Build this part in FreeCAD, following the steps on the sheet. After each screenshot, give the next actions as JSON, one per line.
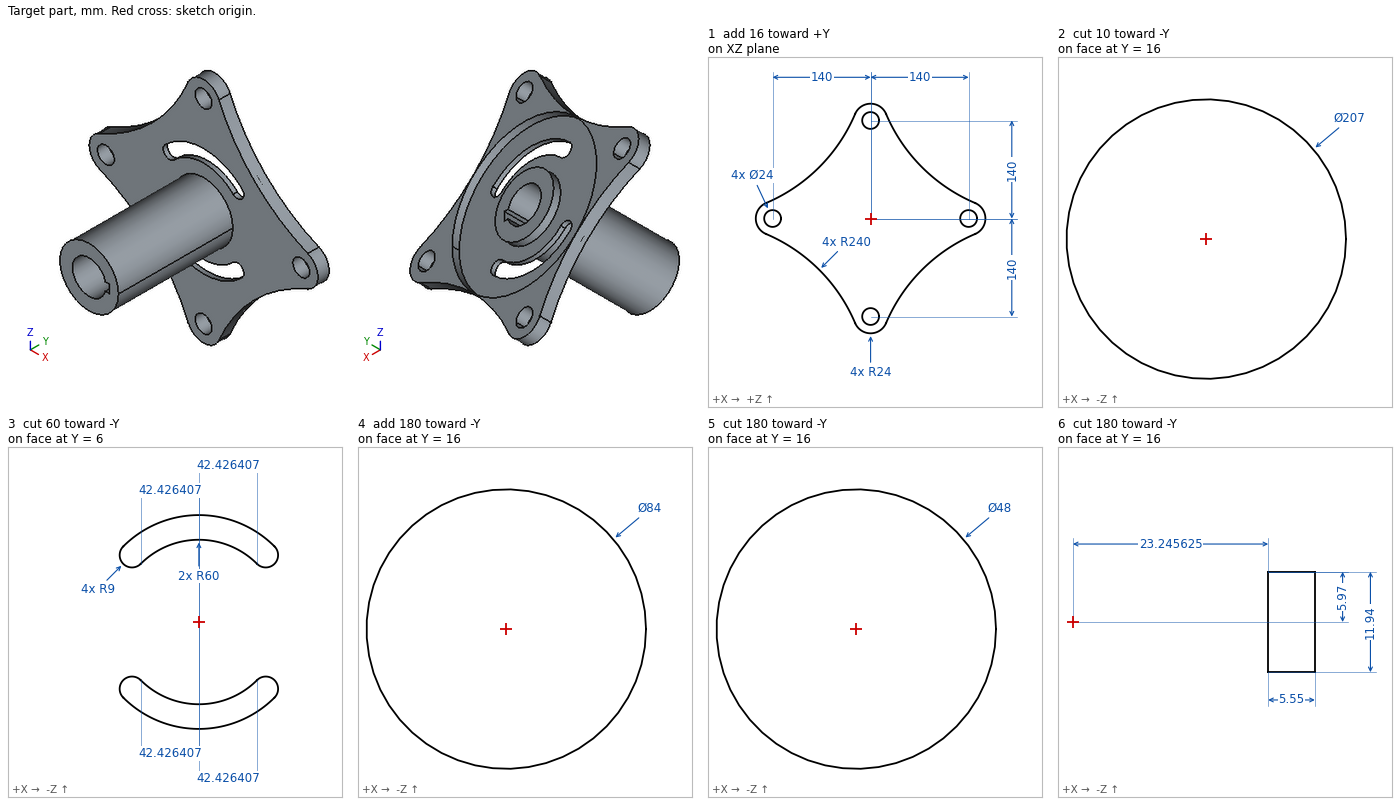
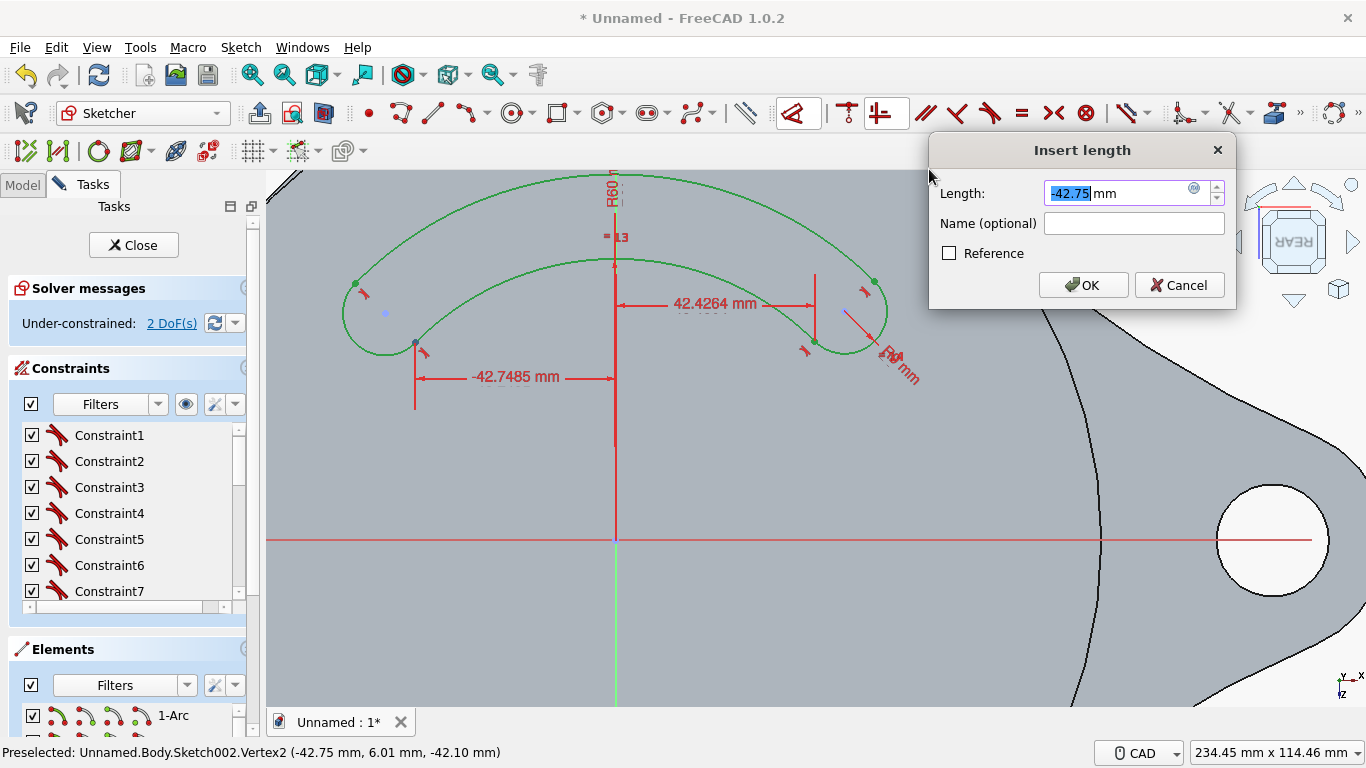
{"action": "type", "text": "-42.426407"}
{"action": "key", "text": "Return"}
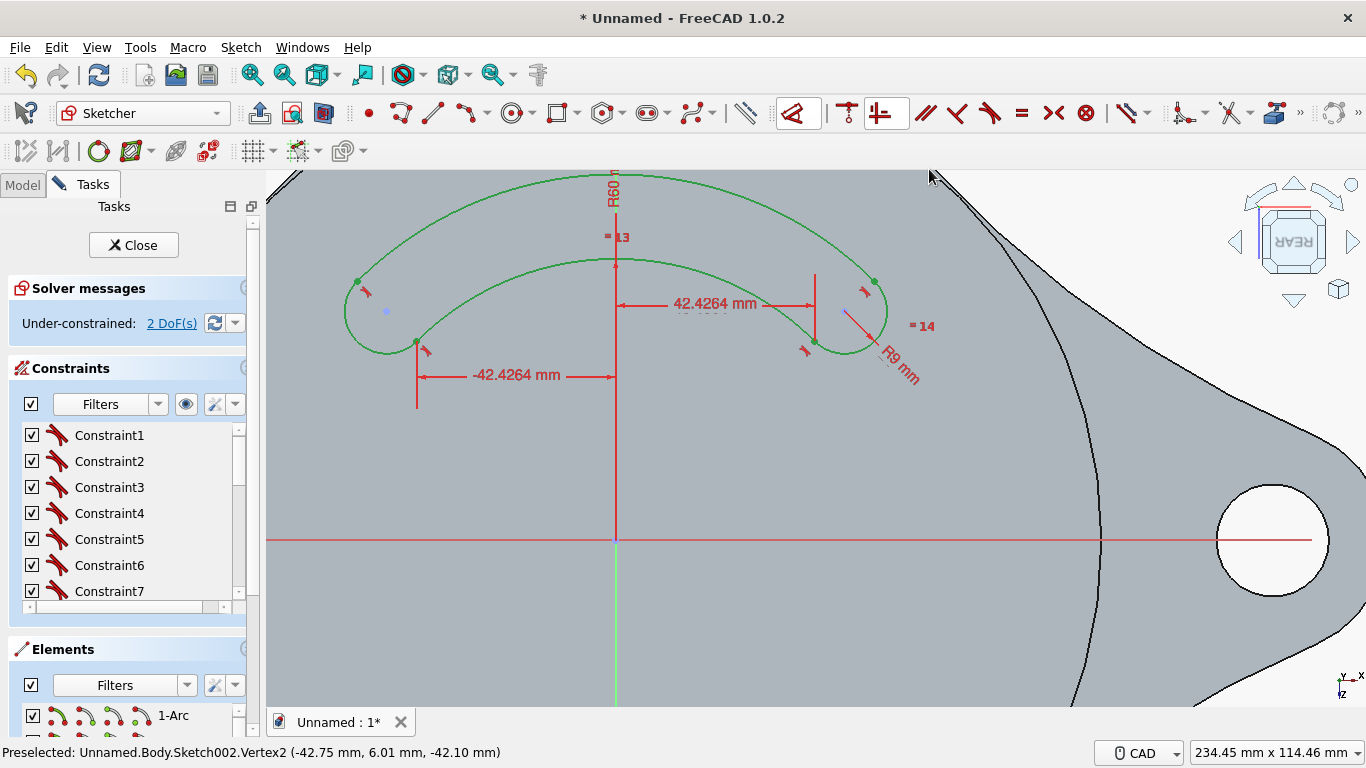
{"action": "scroll", "coordinate": [855, 355], "scroll_direction": "down", "scroll_amount": 4}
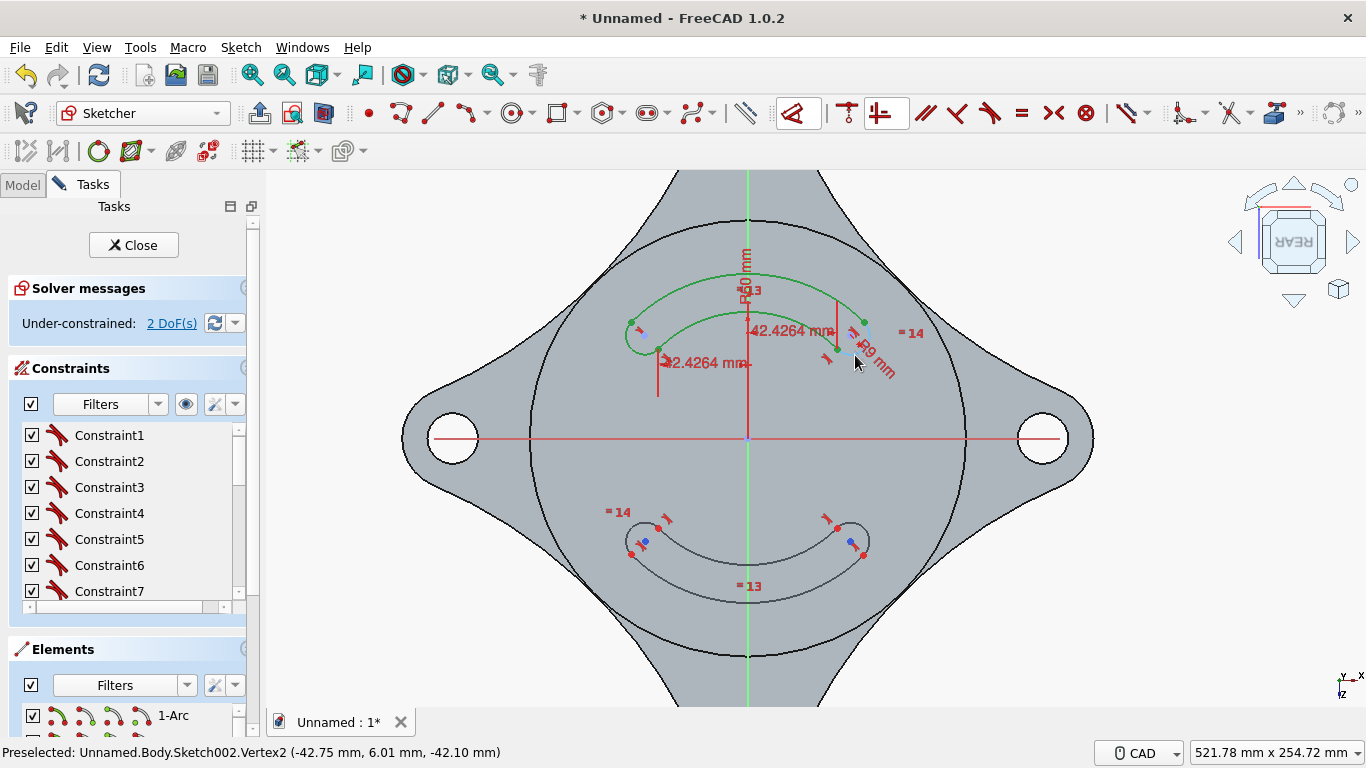
{"action": "left_click", "coordinate": [659, 528]}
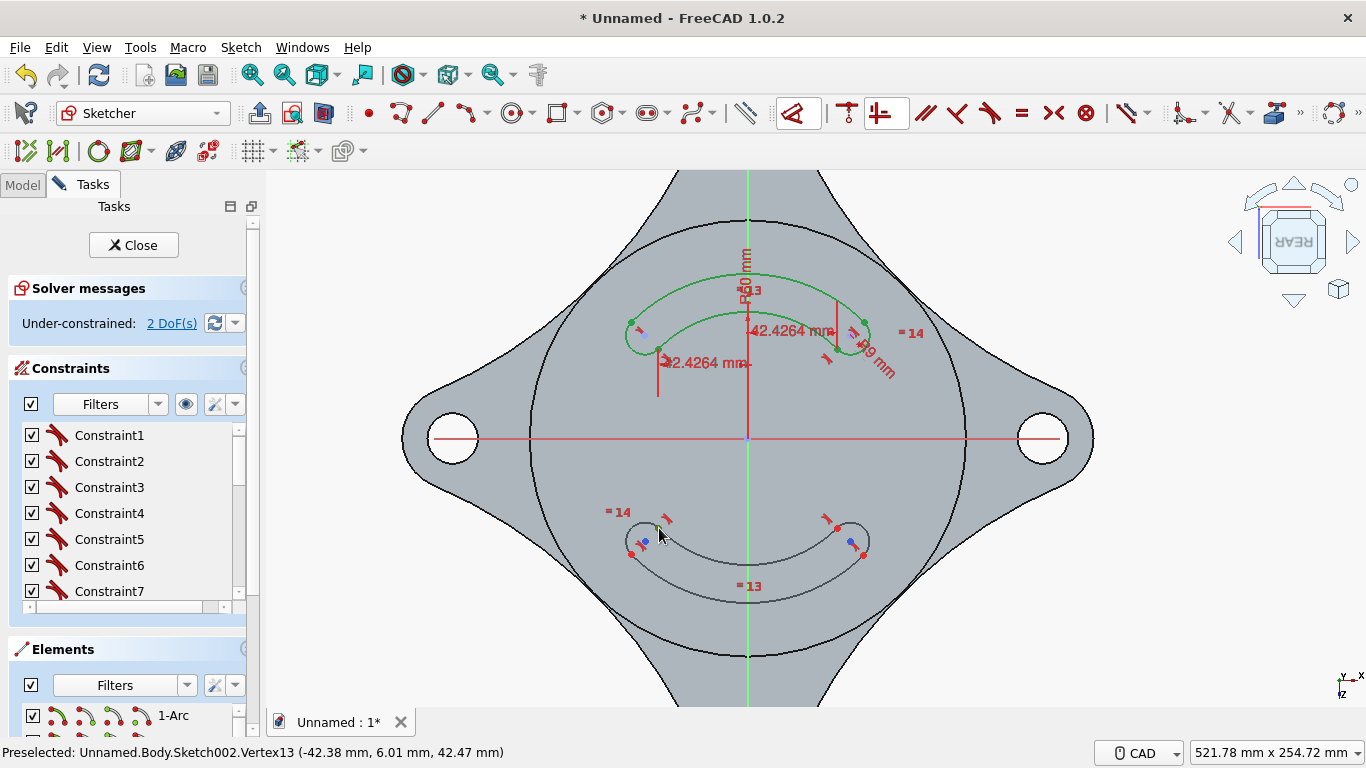
{"action": "left_click", "coordinate": [816, 114]}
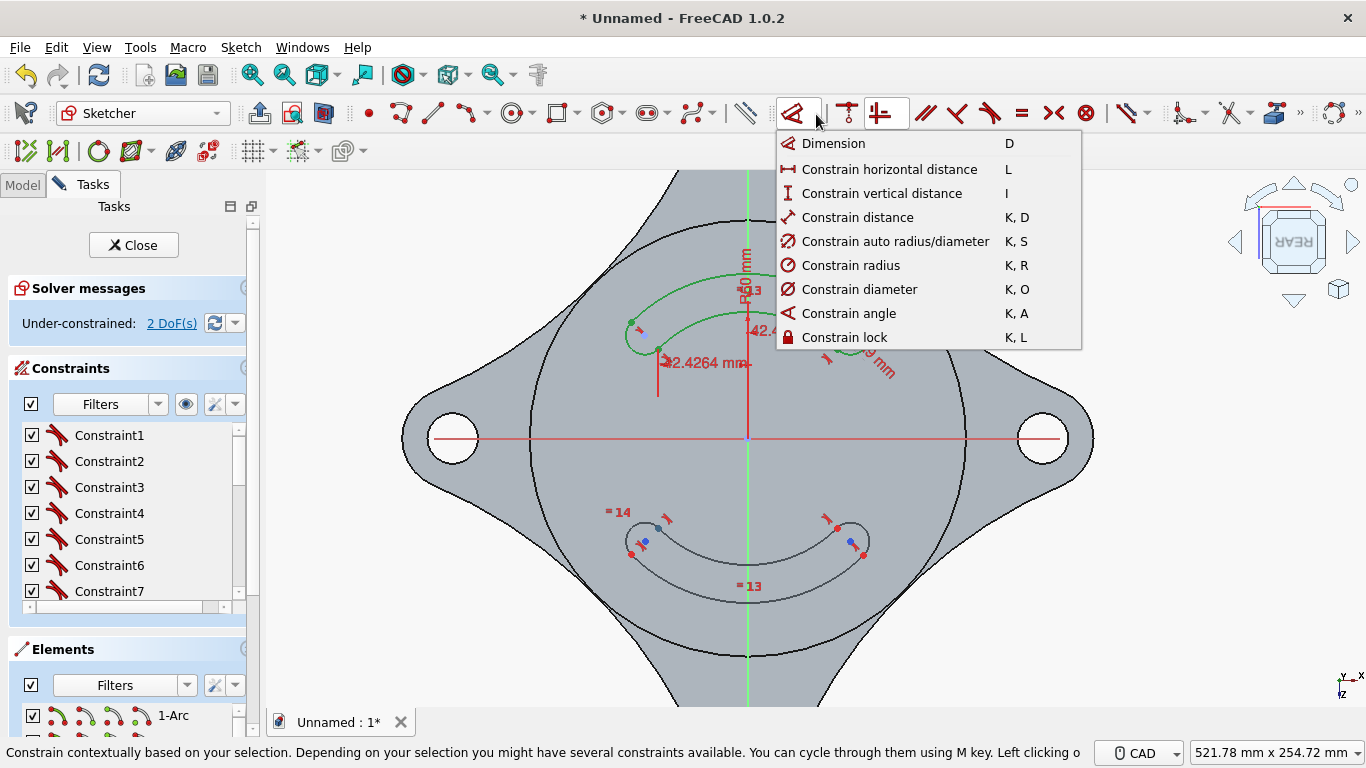
{"action": "left_click", "coordinate": [929, 169]}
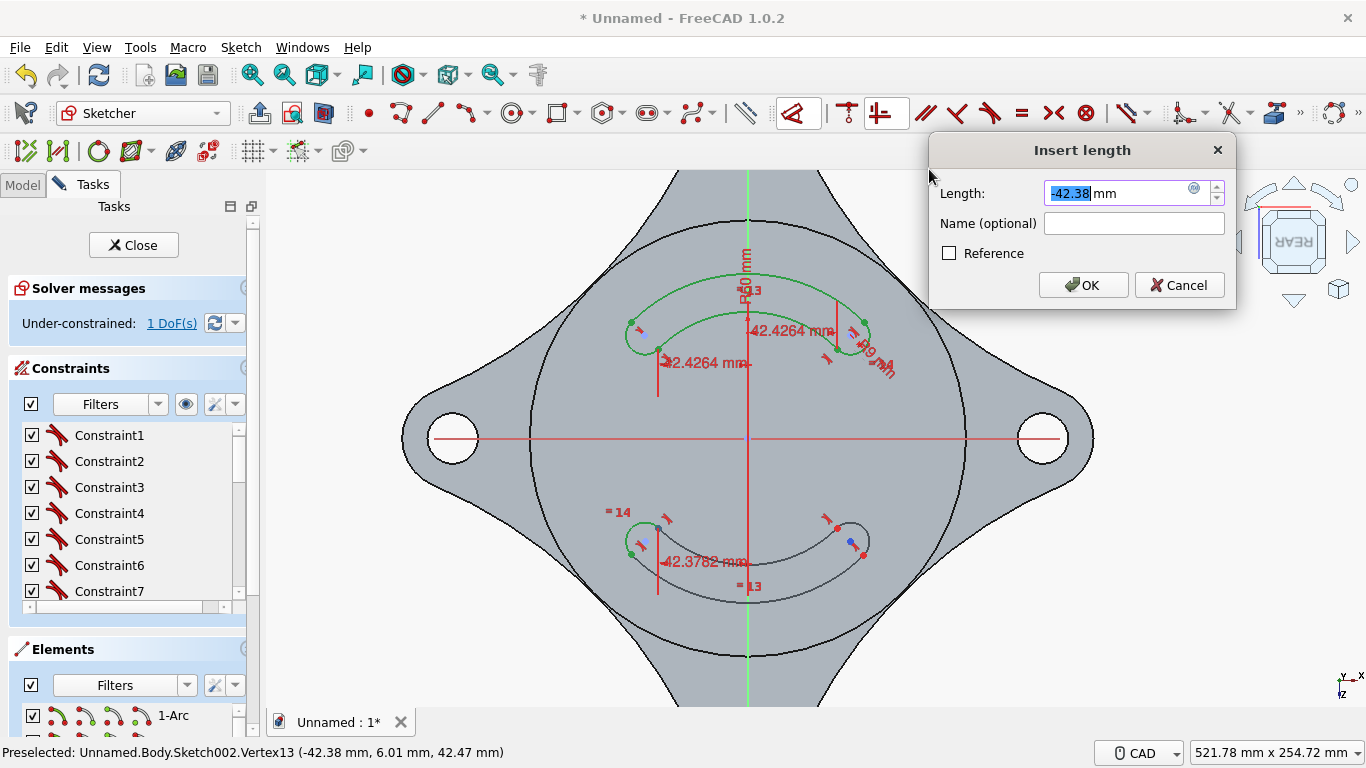
{"action": "type", "text": "-42.426407"}
{"action": "key", "text": "Return"}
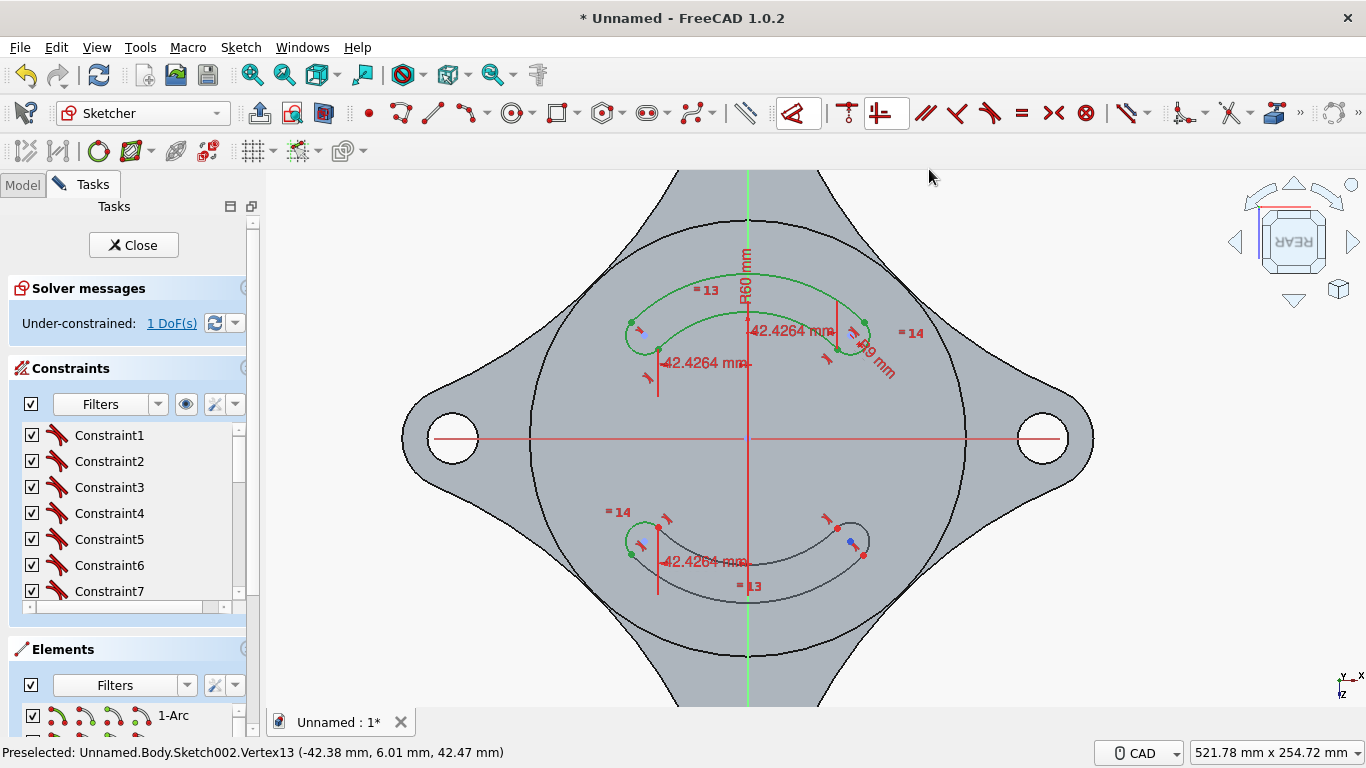
{"action": "left_click", "coordinate": [837, 528]}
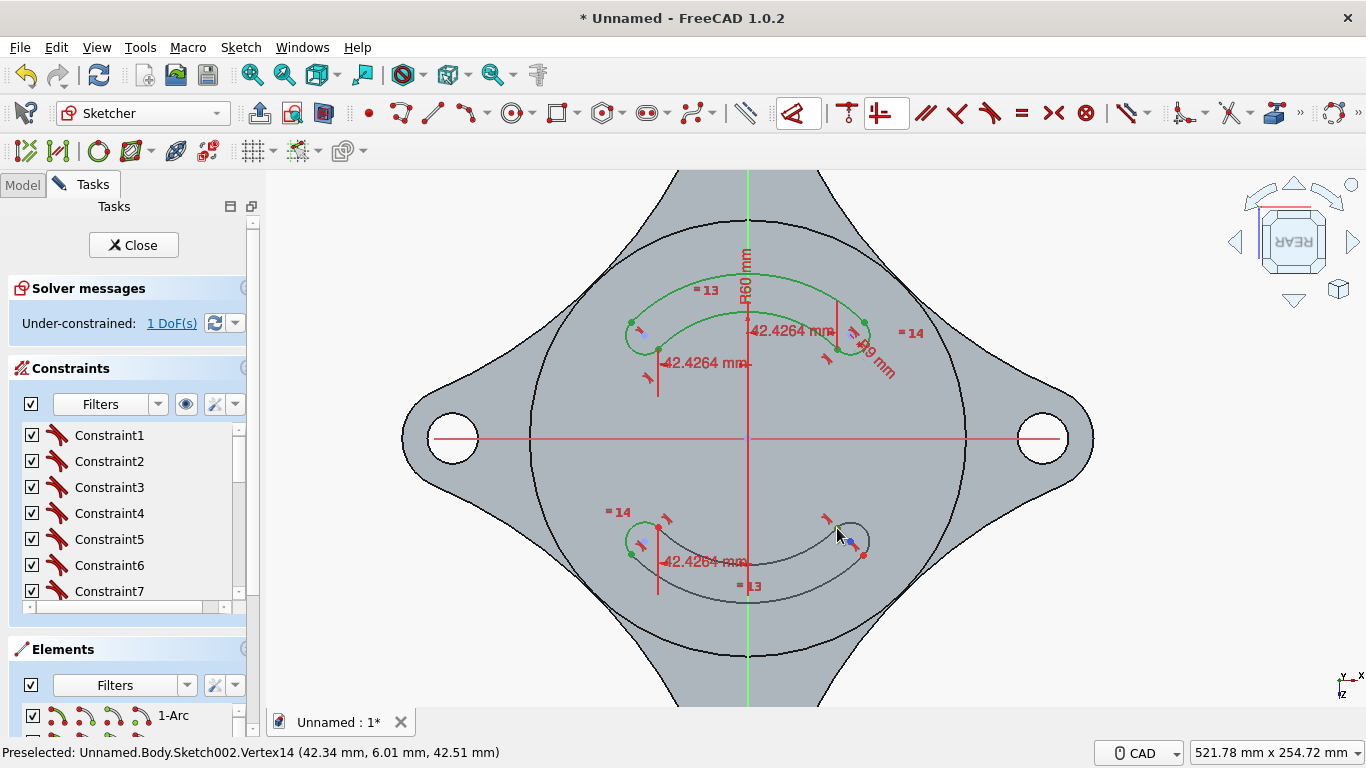
{"action": "key", "text": "l"}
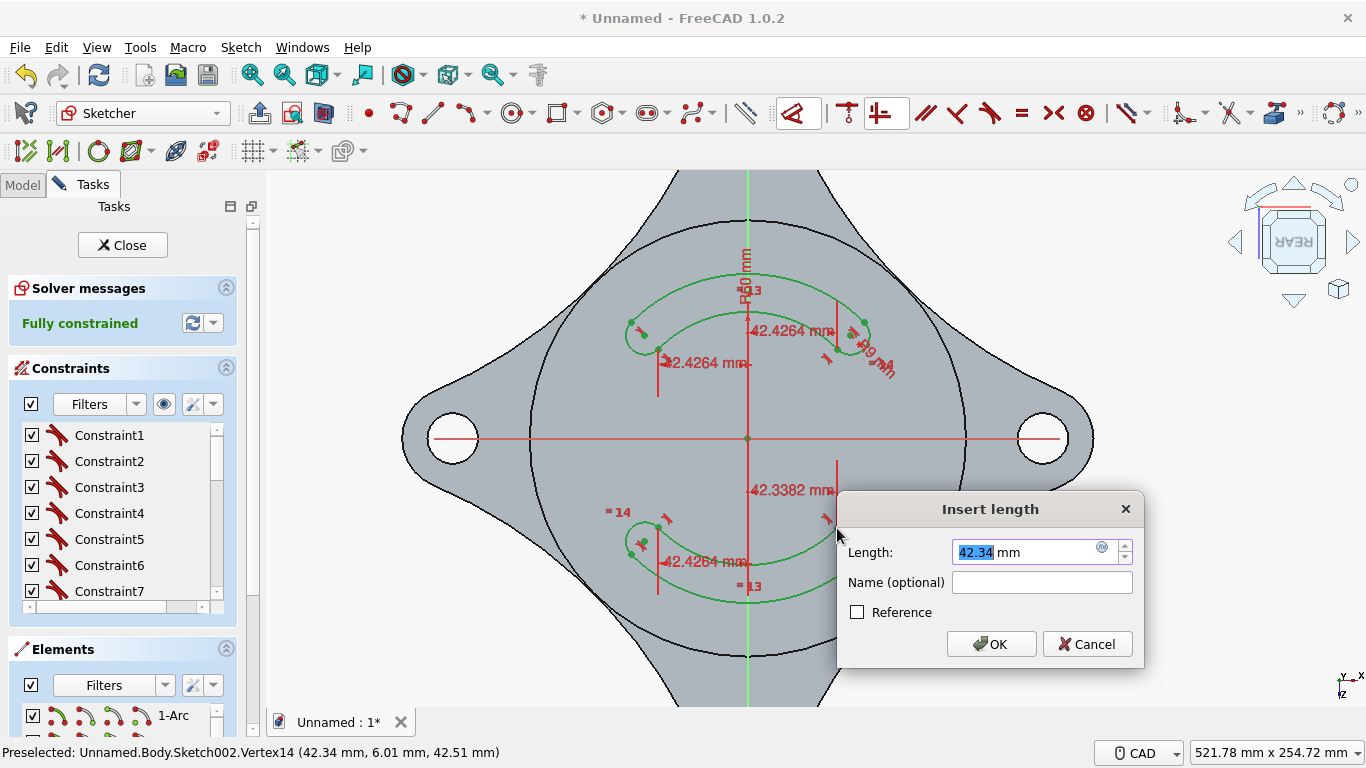
{"action": "type", "text": "42.426407"}
{"action": "key", "text": "Return"}